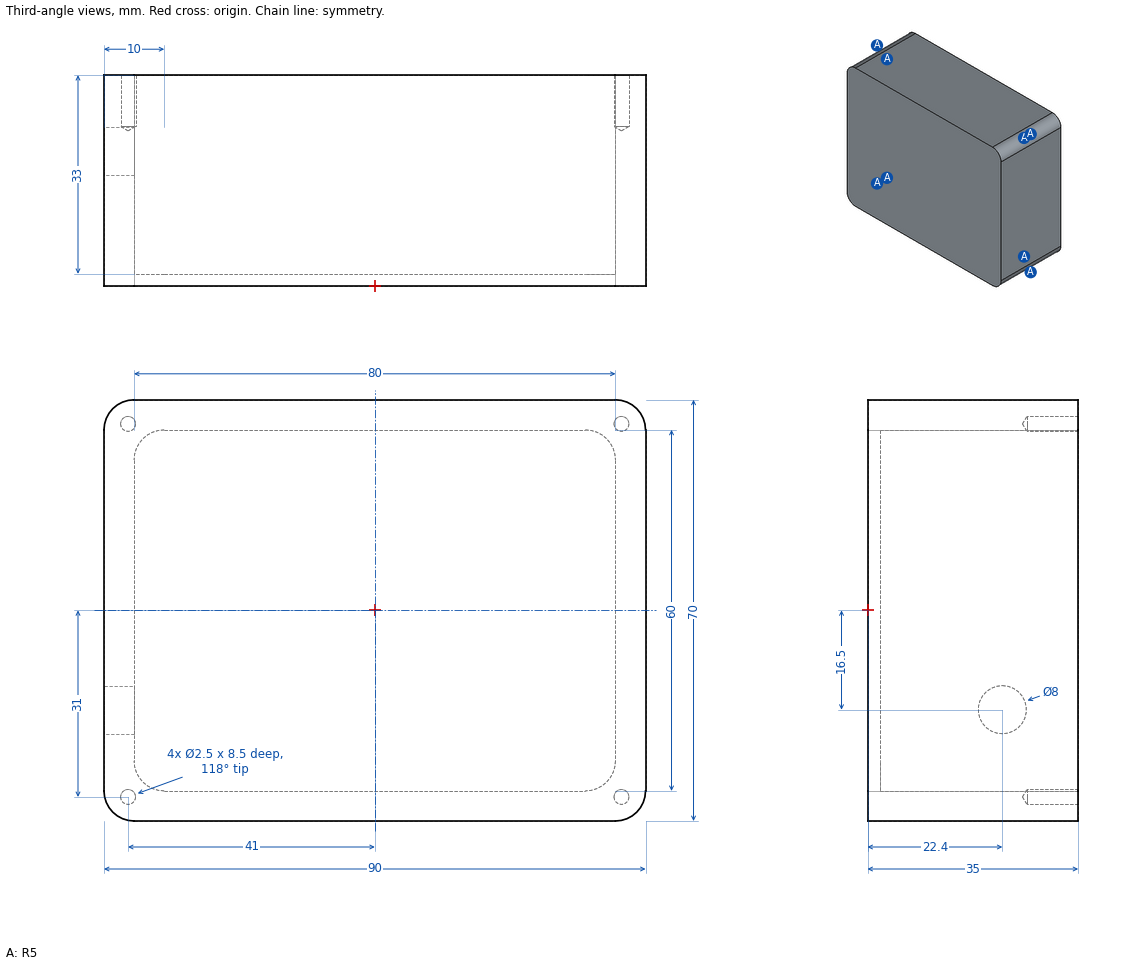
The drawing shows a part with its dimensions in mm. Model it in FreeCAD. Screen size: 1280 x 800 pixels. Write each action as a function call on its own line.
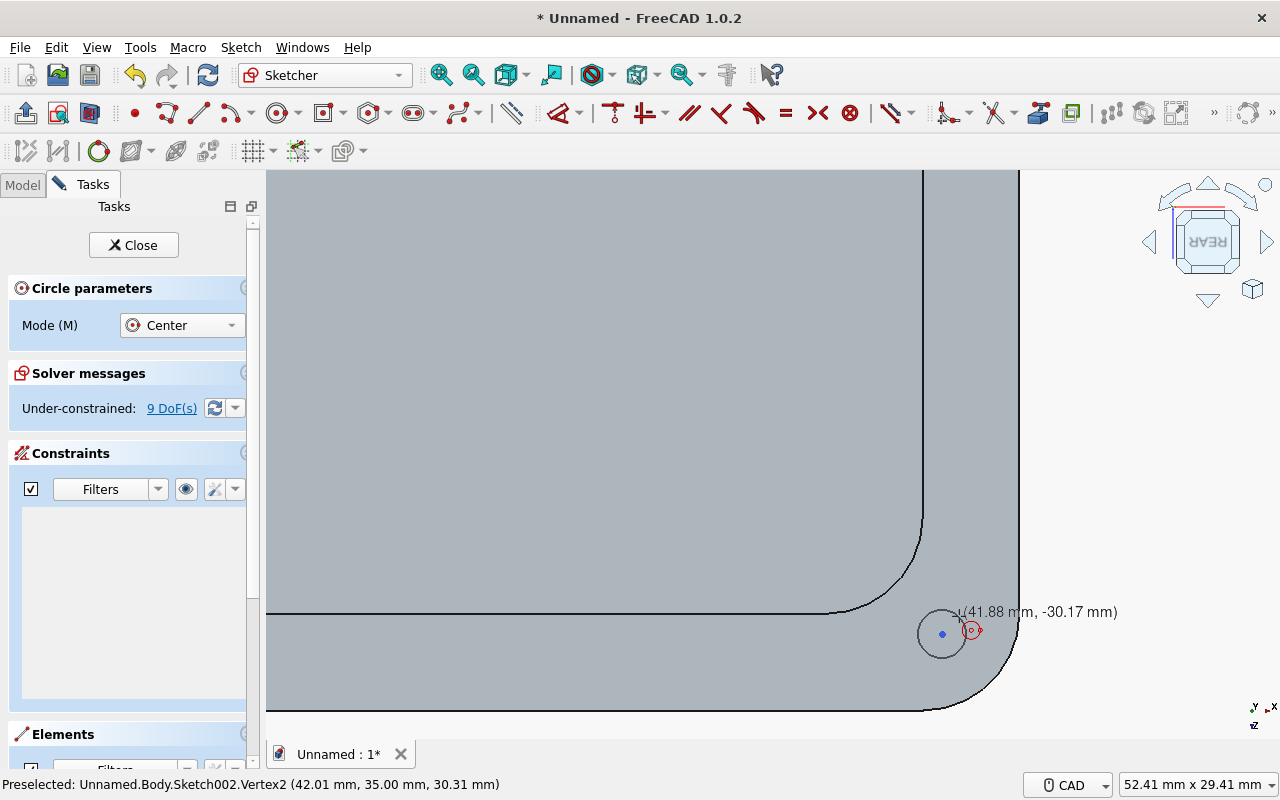
scroll(944, 636, down, 6)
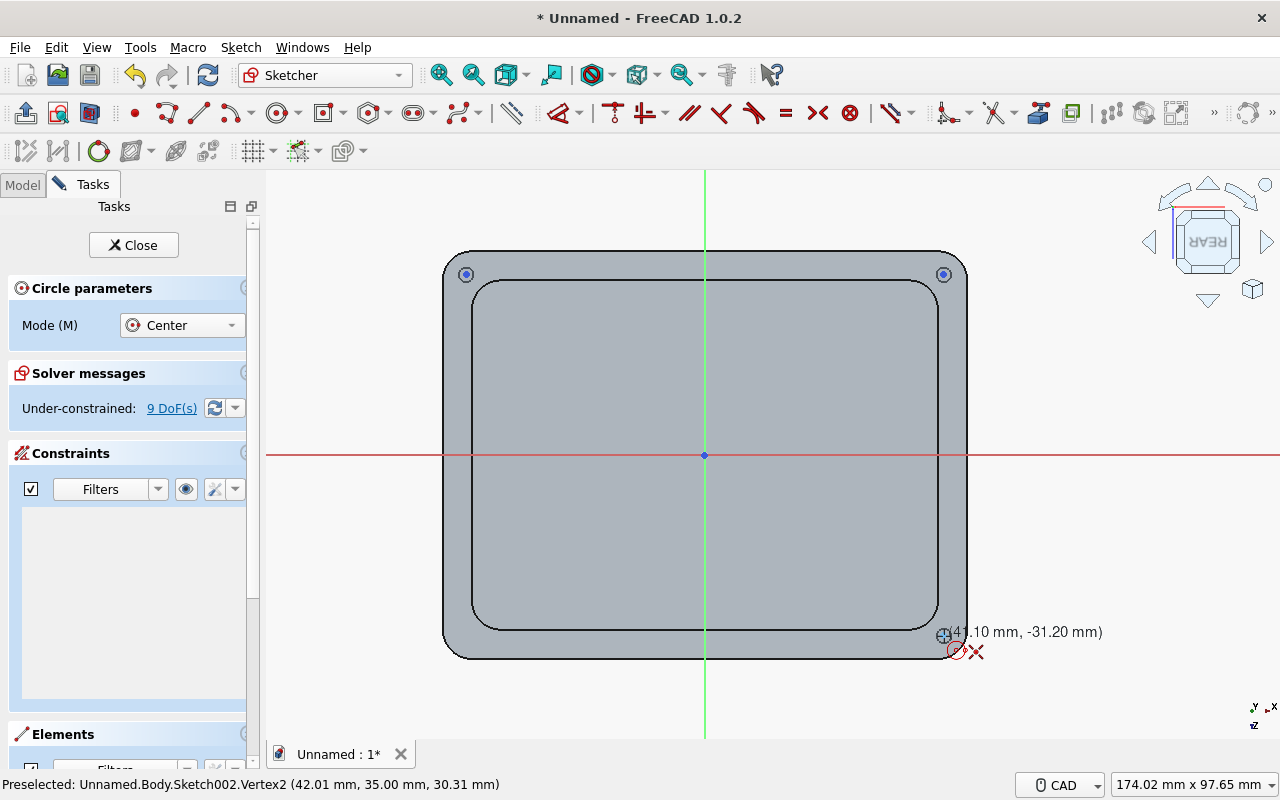
scroll(466, 636, up, 6)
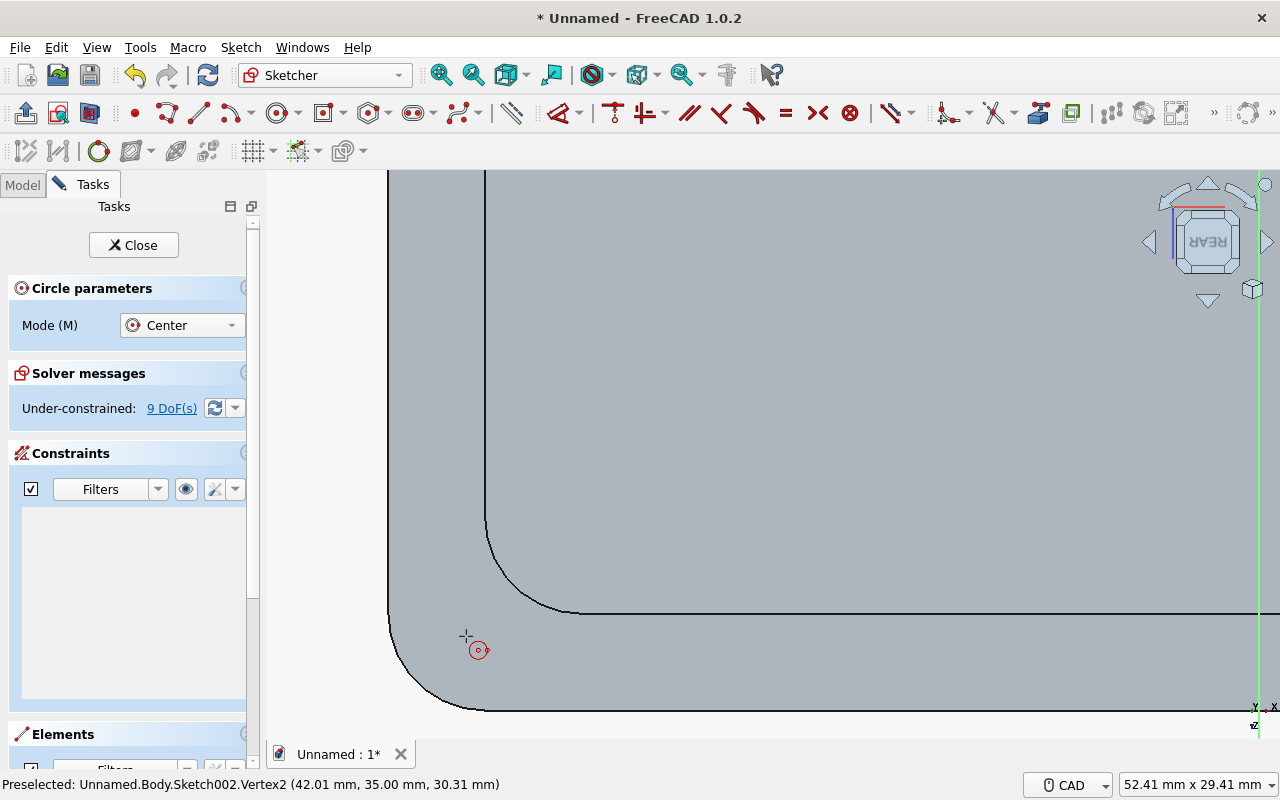
click(466, 633)
click(483, 616)
key(Escape)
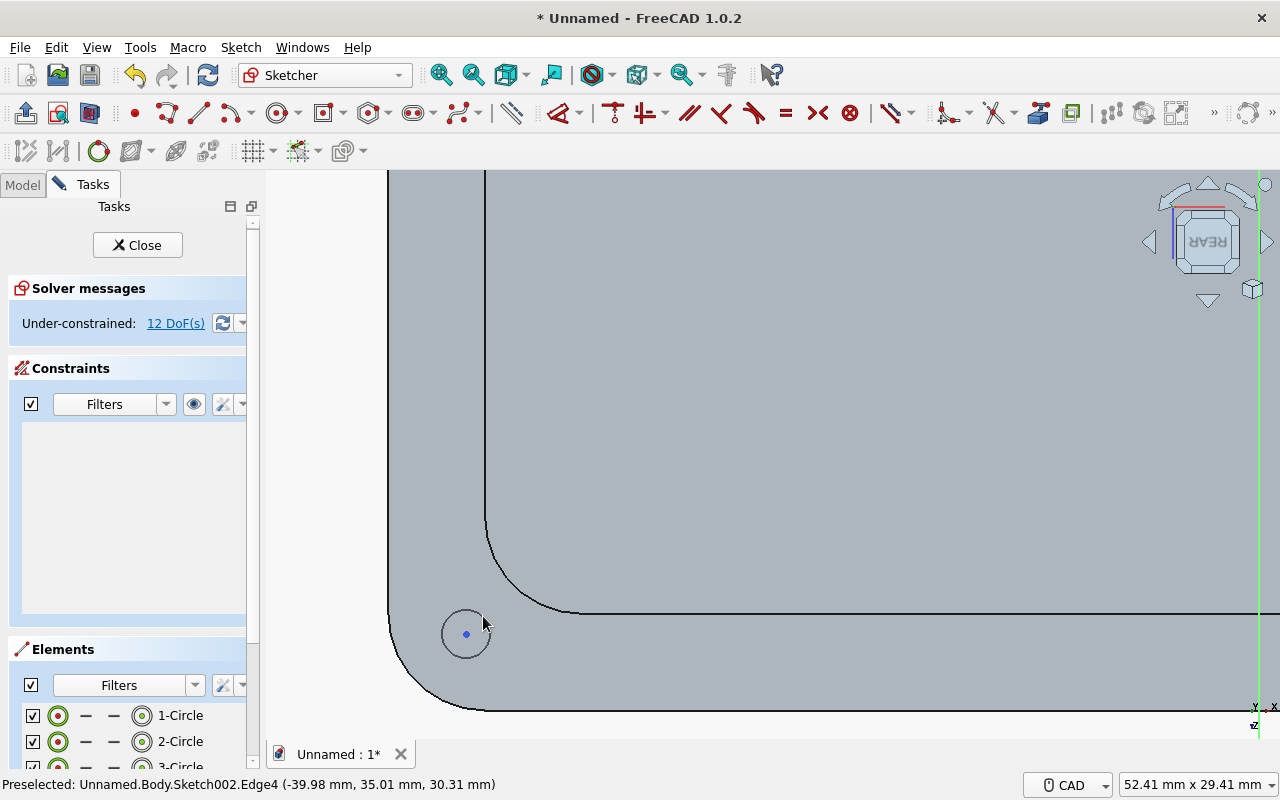
scroll(466, 636, down, 6)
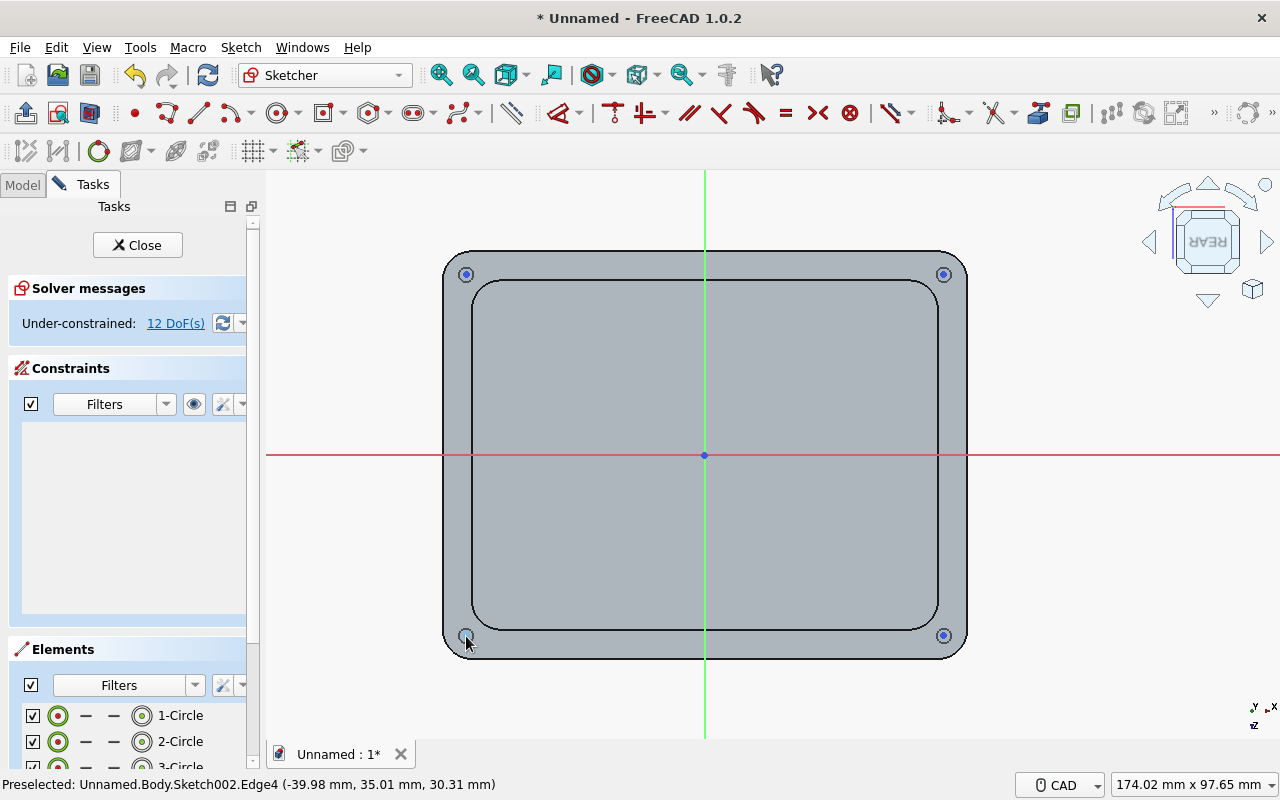
scroll(471, 270, up, 4)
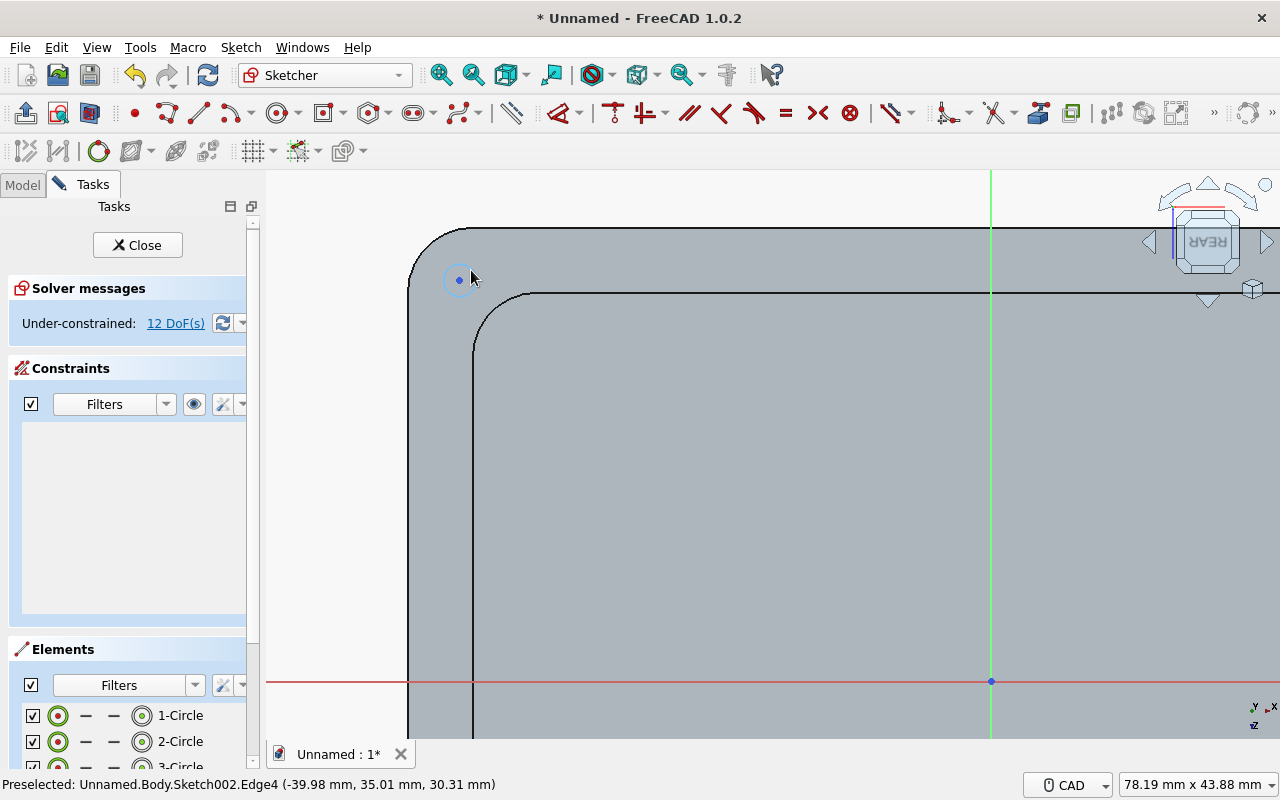
click(471, 269)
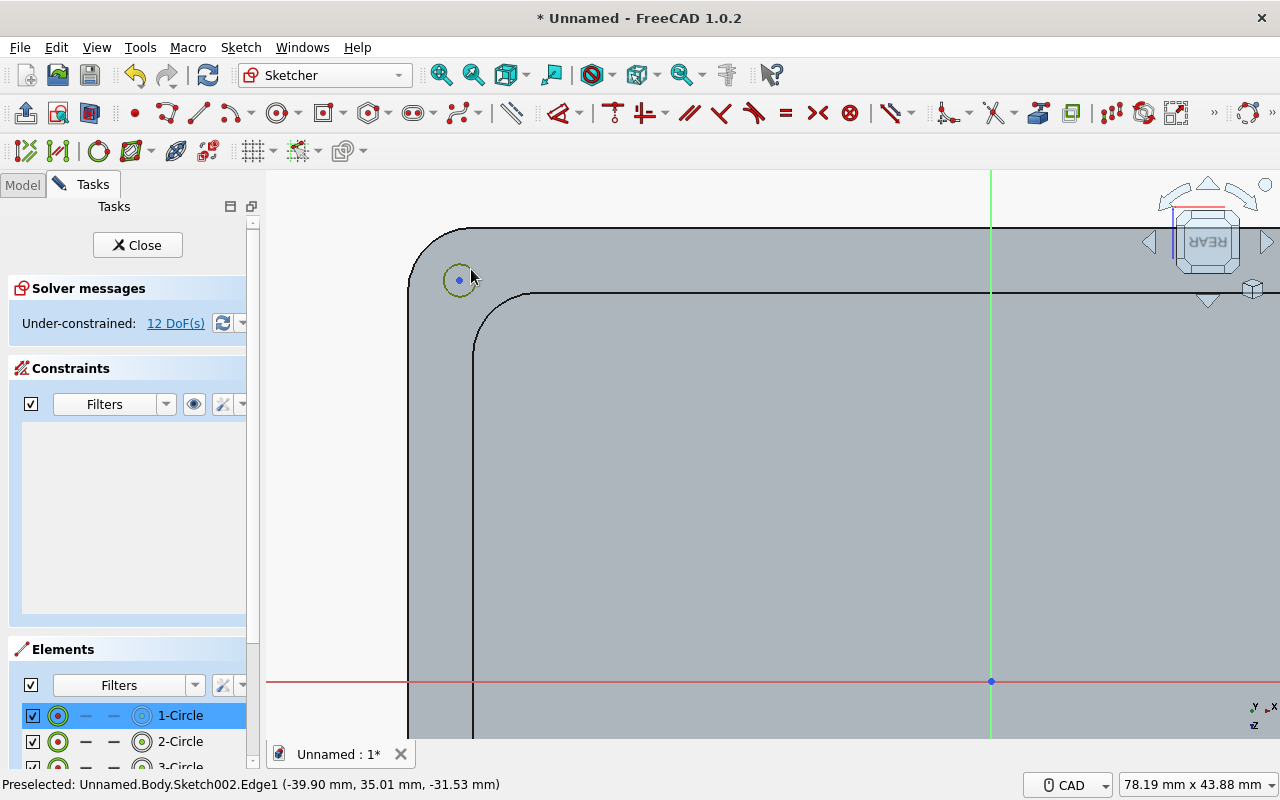
scroll(470, 269, down, 4)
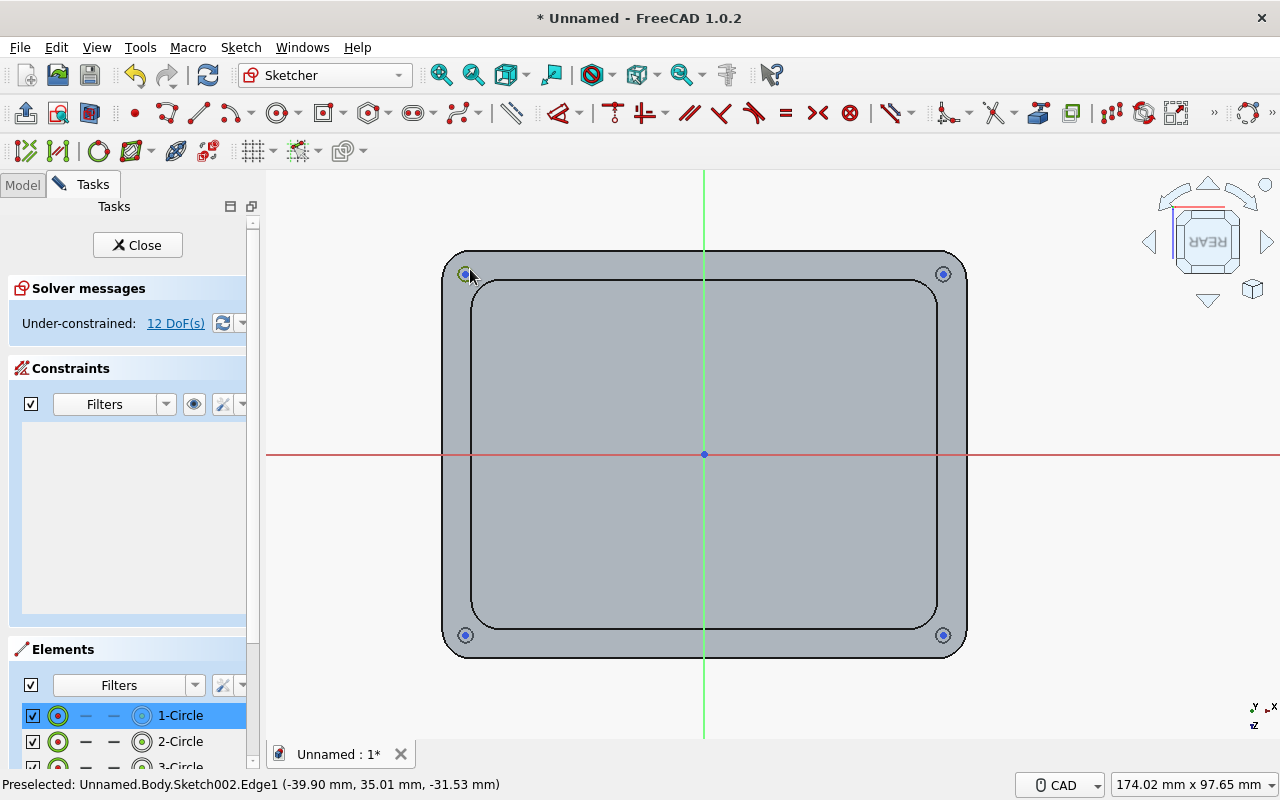
scroll(948, 269, up, 4)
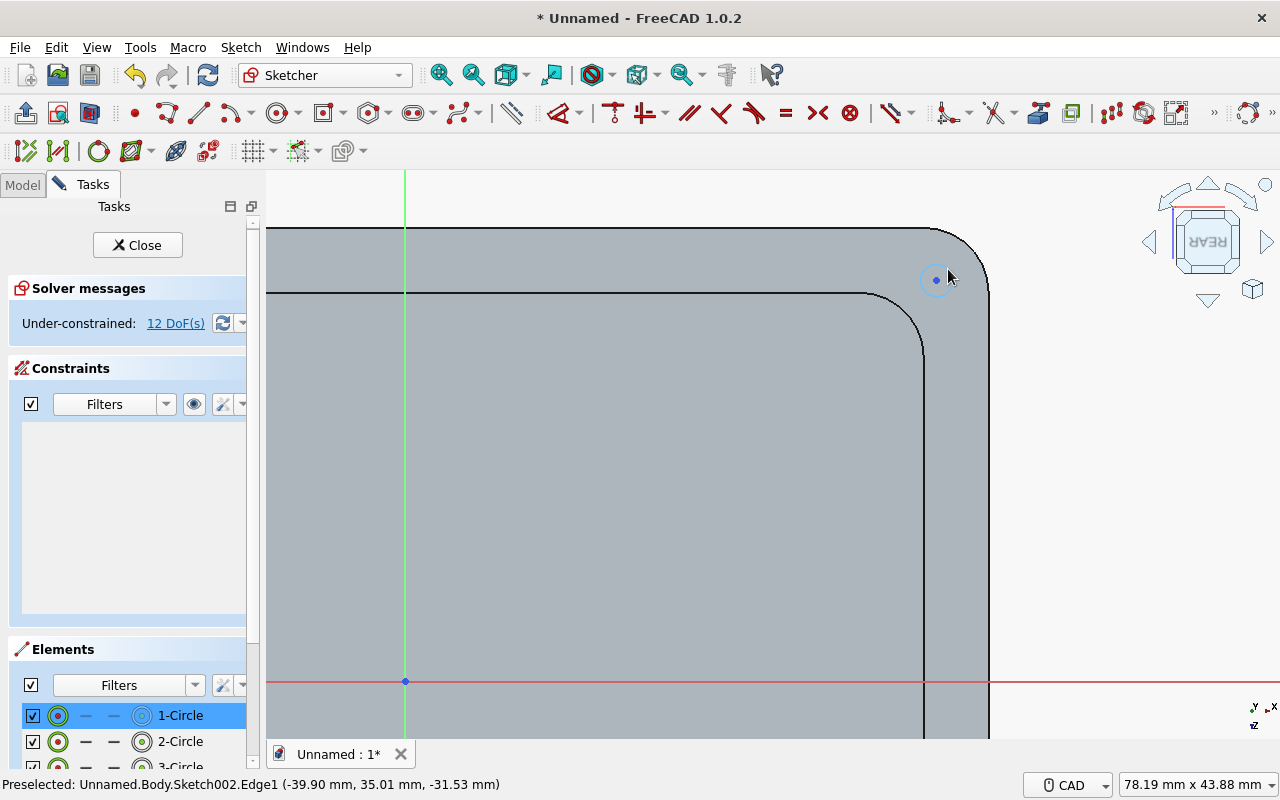
click(948, 269)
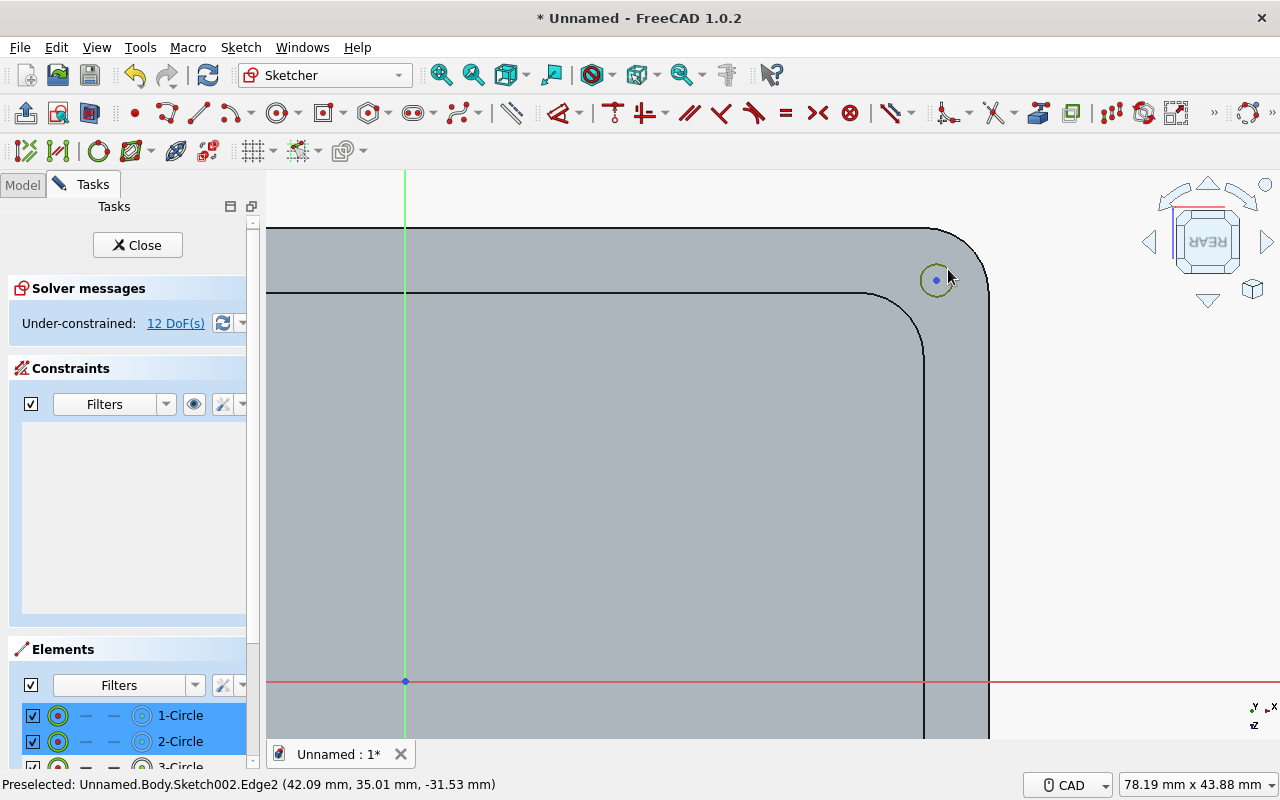
scroll(949, 269, down, 4)